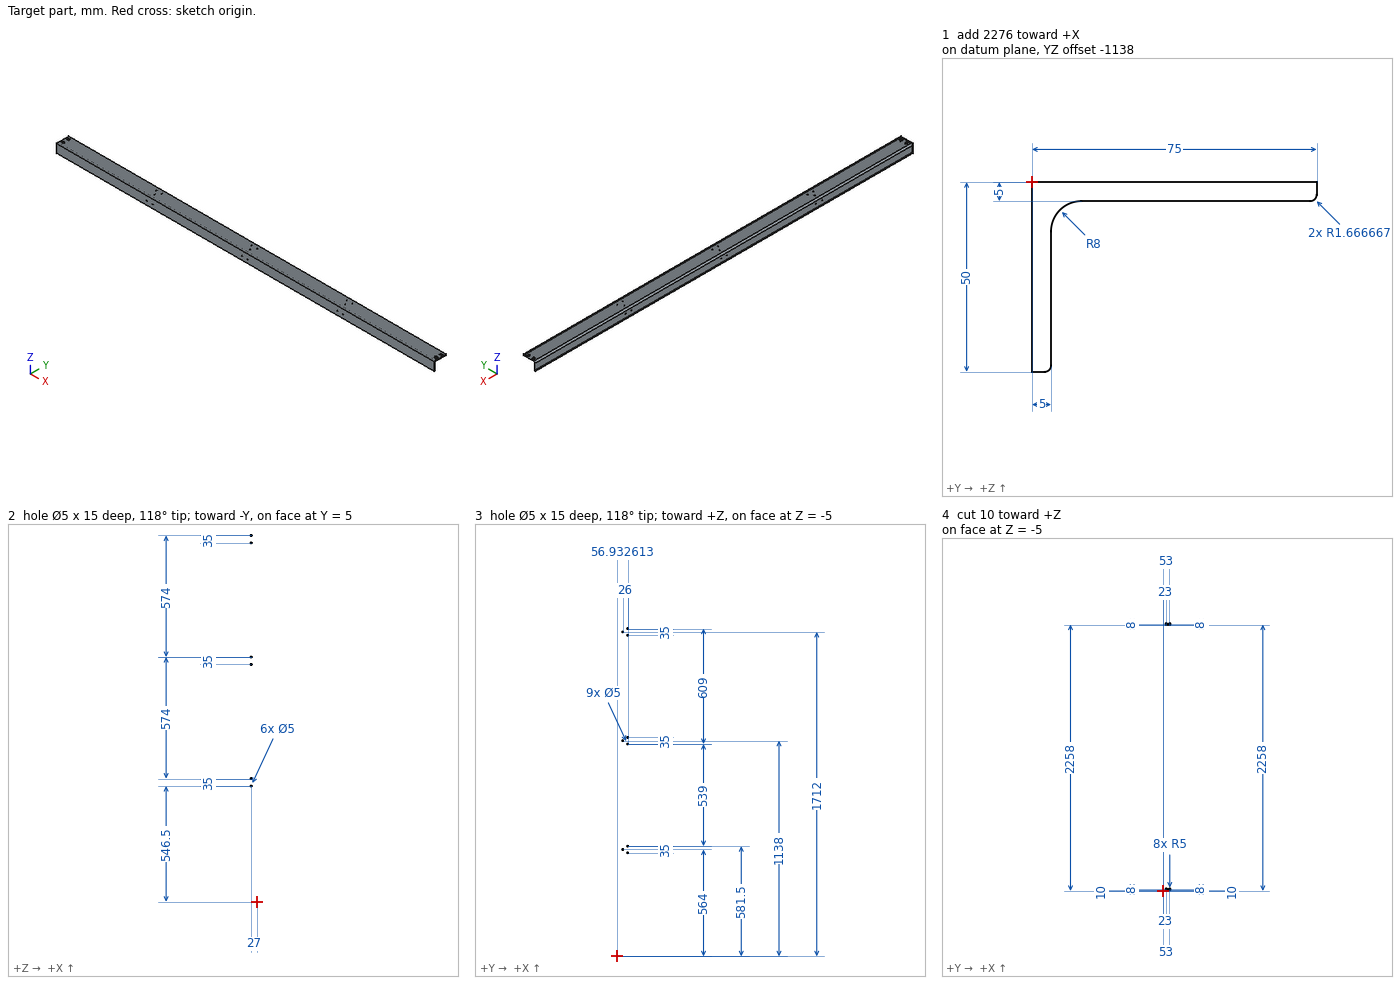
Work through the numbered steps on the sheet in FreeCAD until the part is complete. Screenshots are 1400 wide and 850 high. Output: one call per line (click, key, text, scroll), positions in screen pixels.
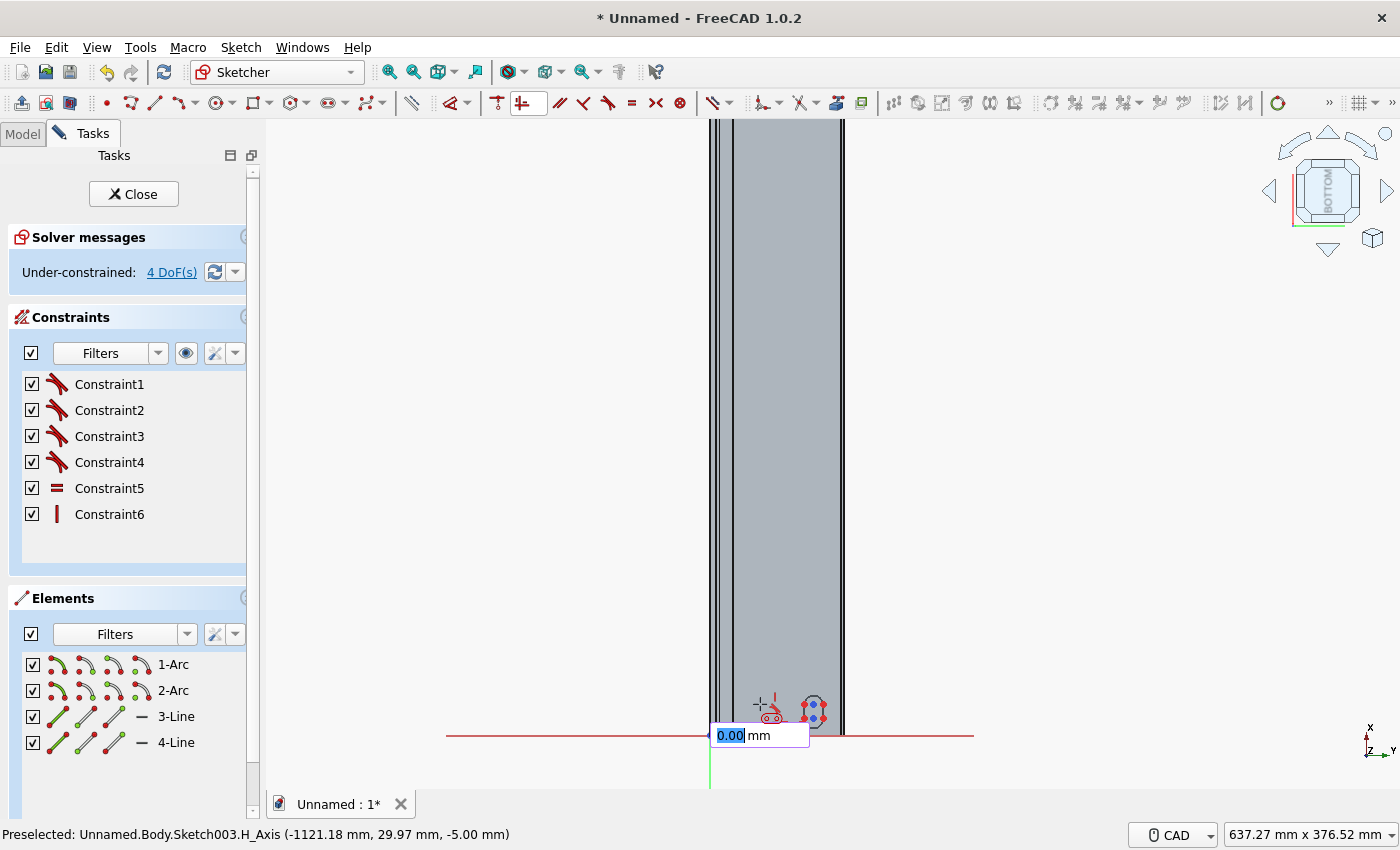
scroll(769, 711, up, 3)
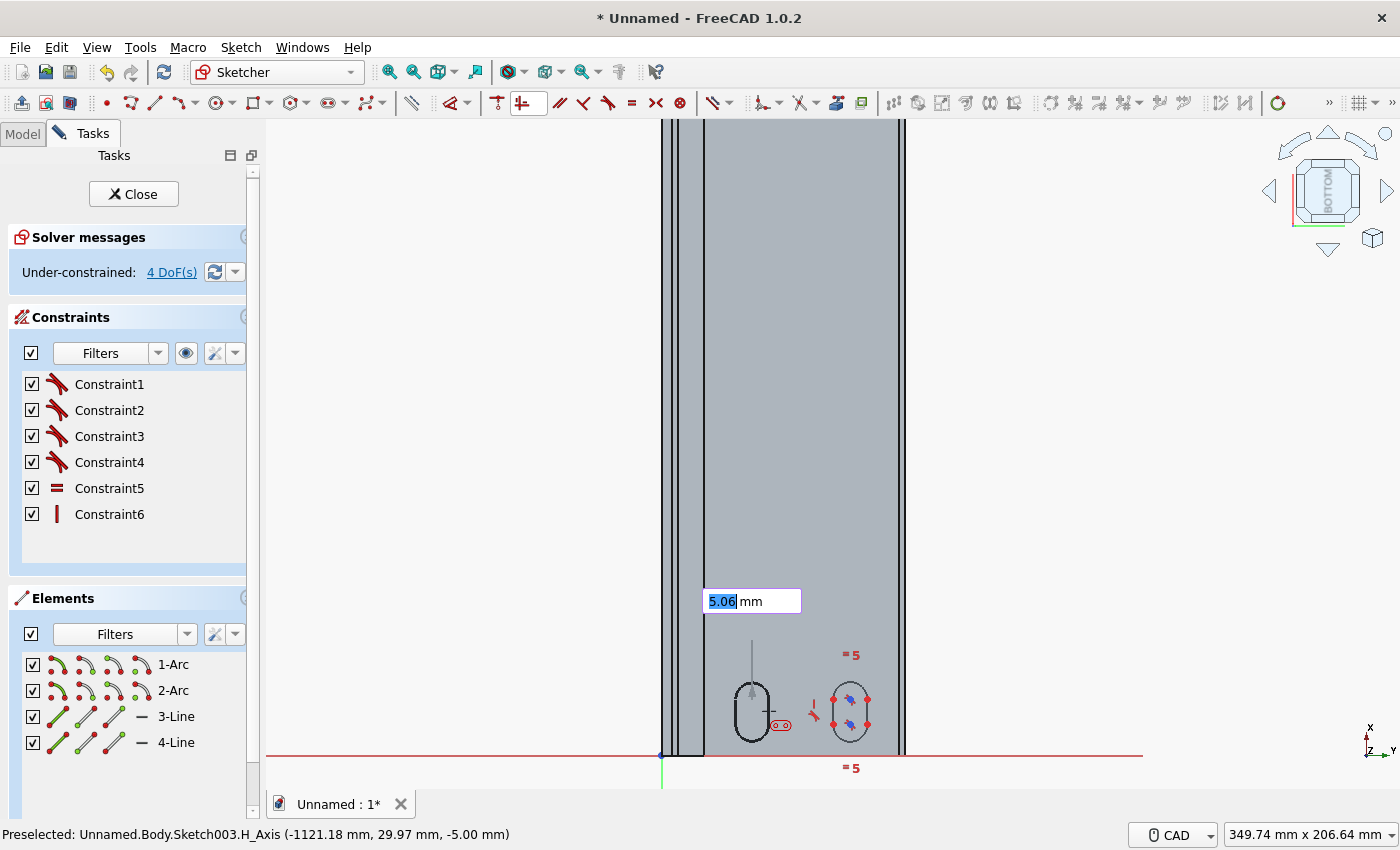
click(769, 710)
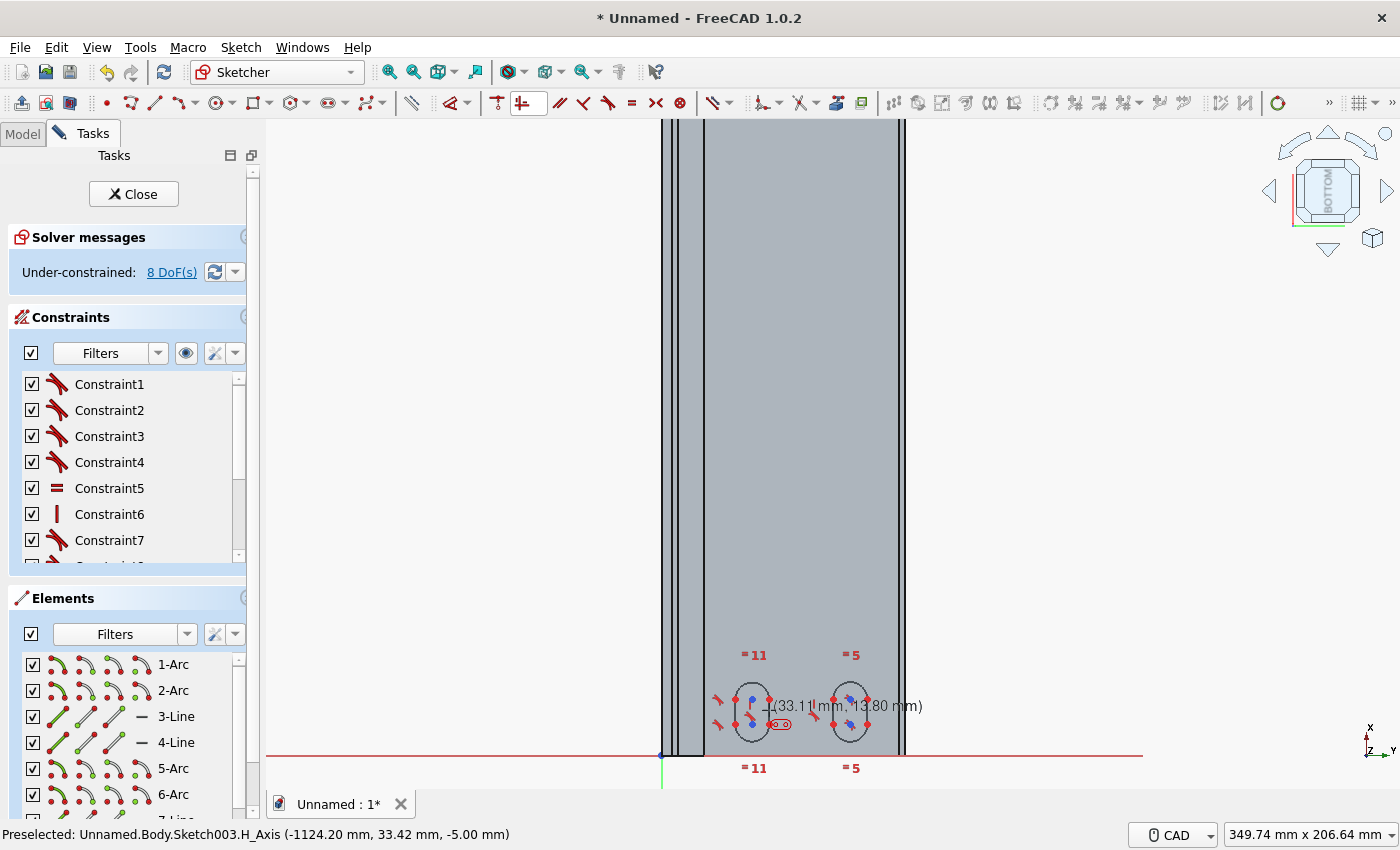
scroll(765, 673, down, 14)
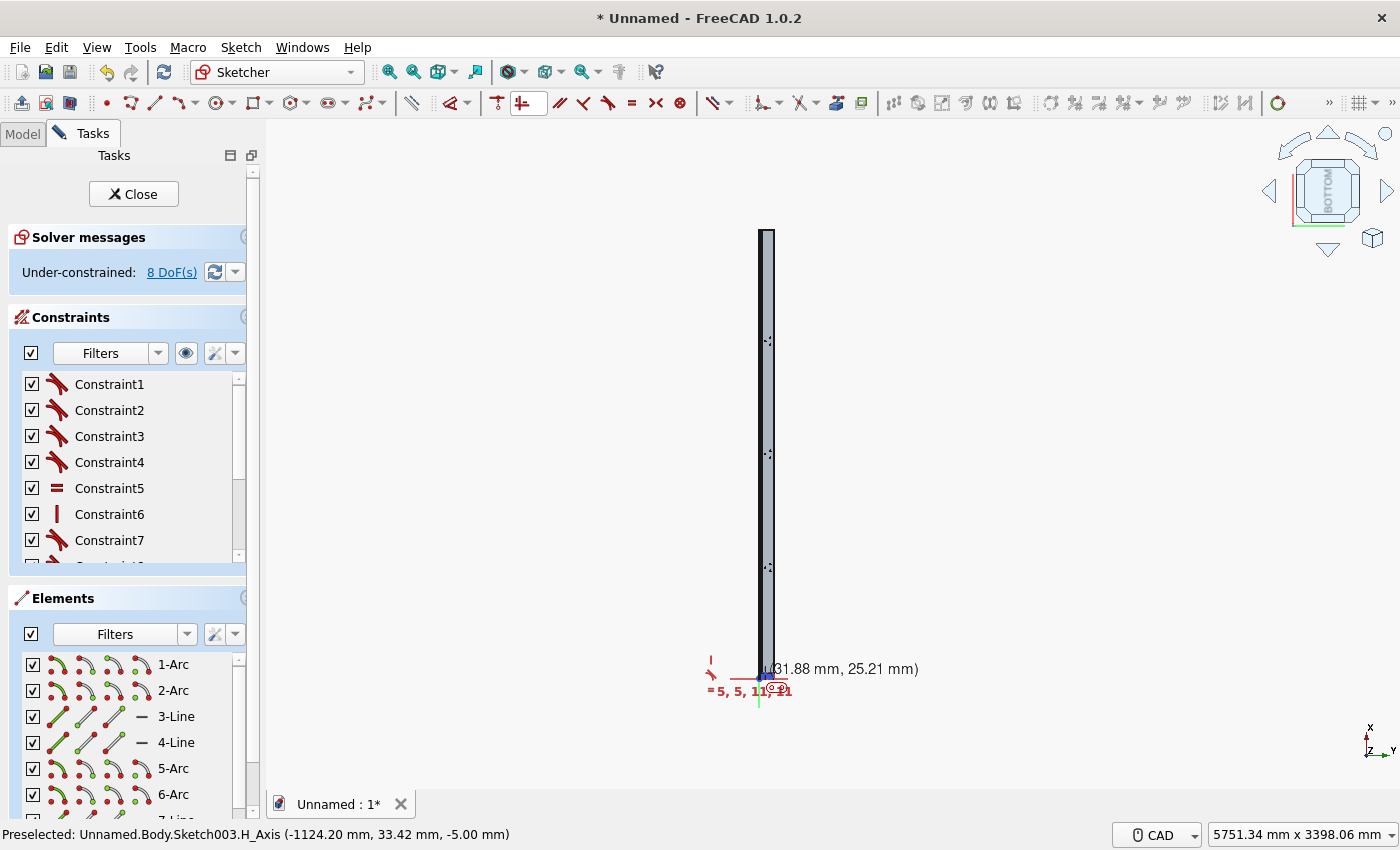
scroll(771, 234, up, 16)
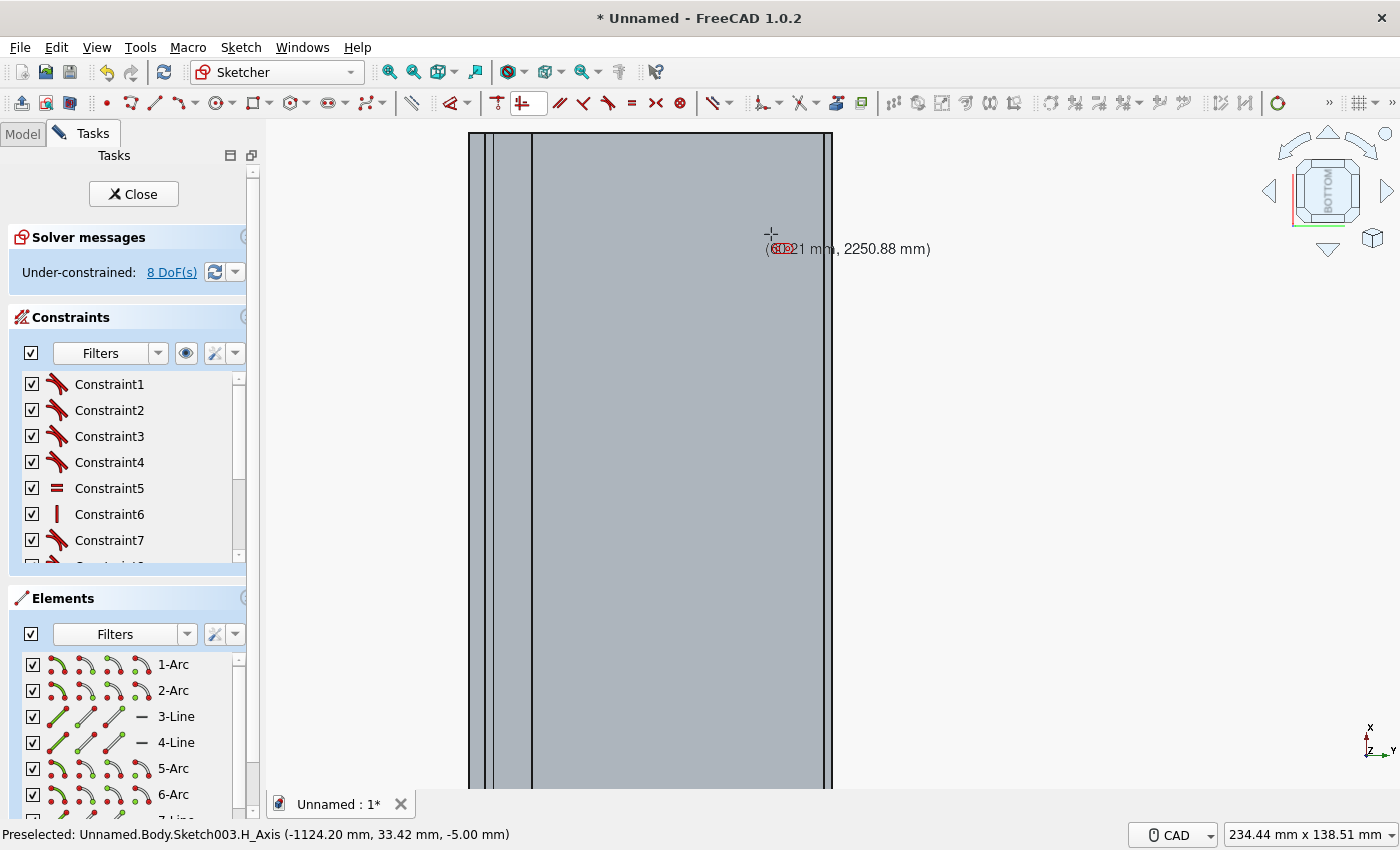
scroll(772, 182, down, 15)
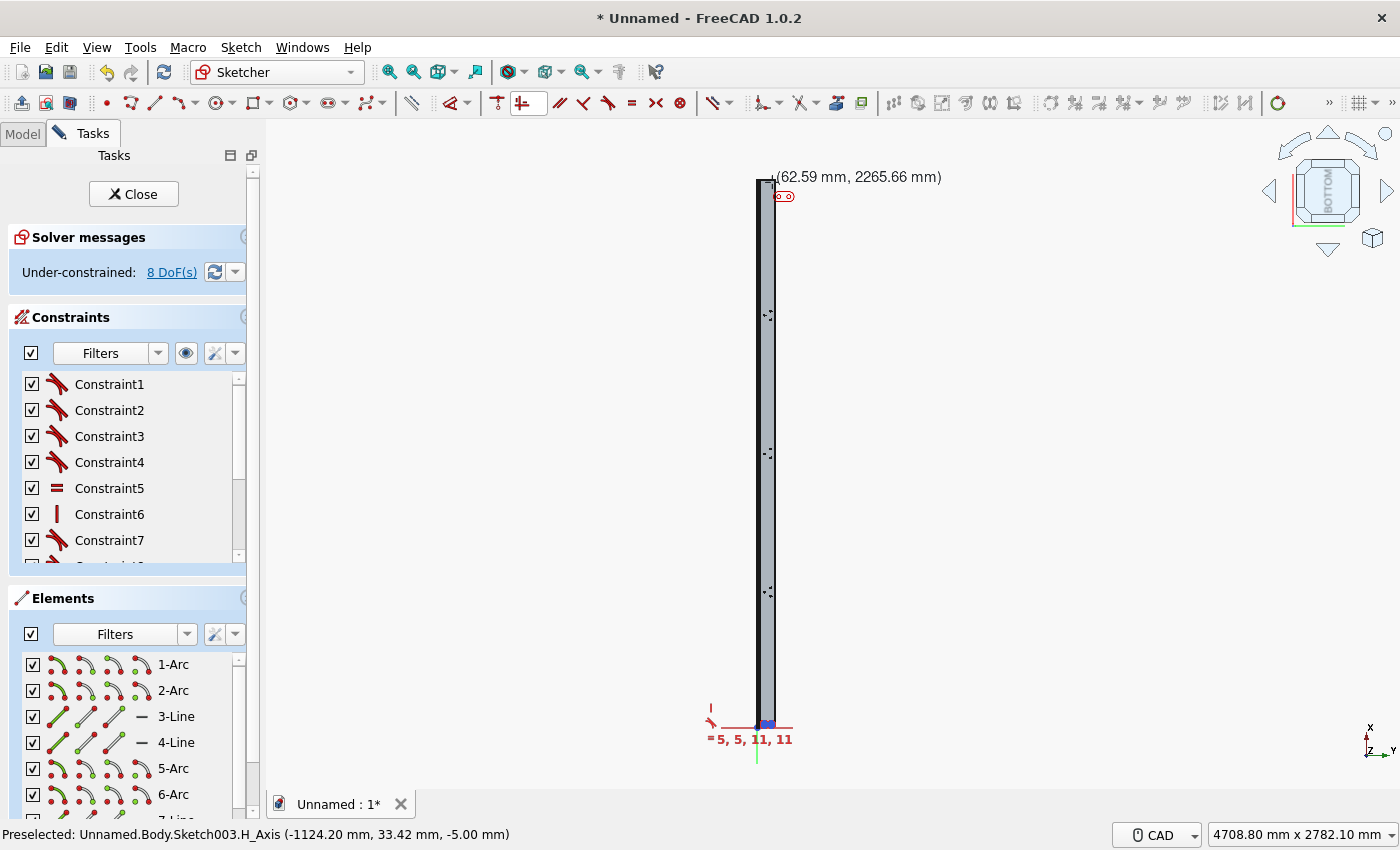
click(771, 184)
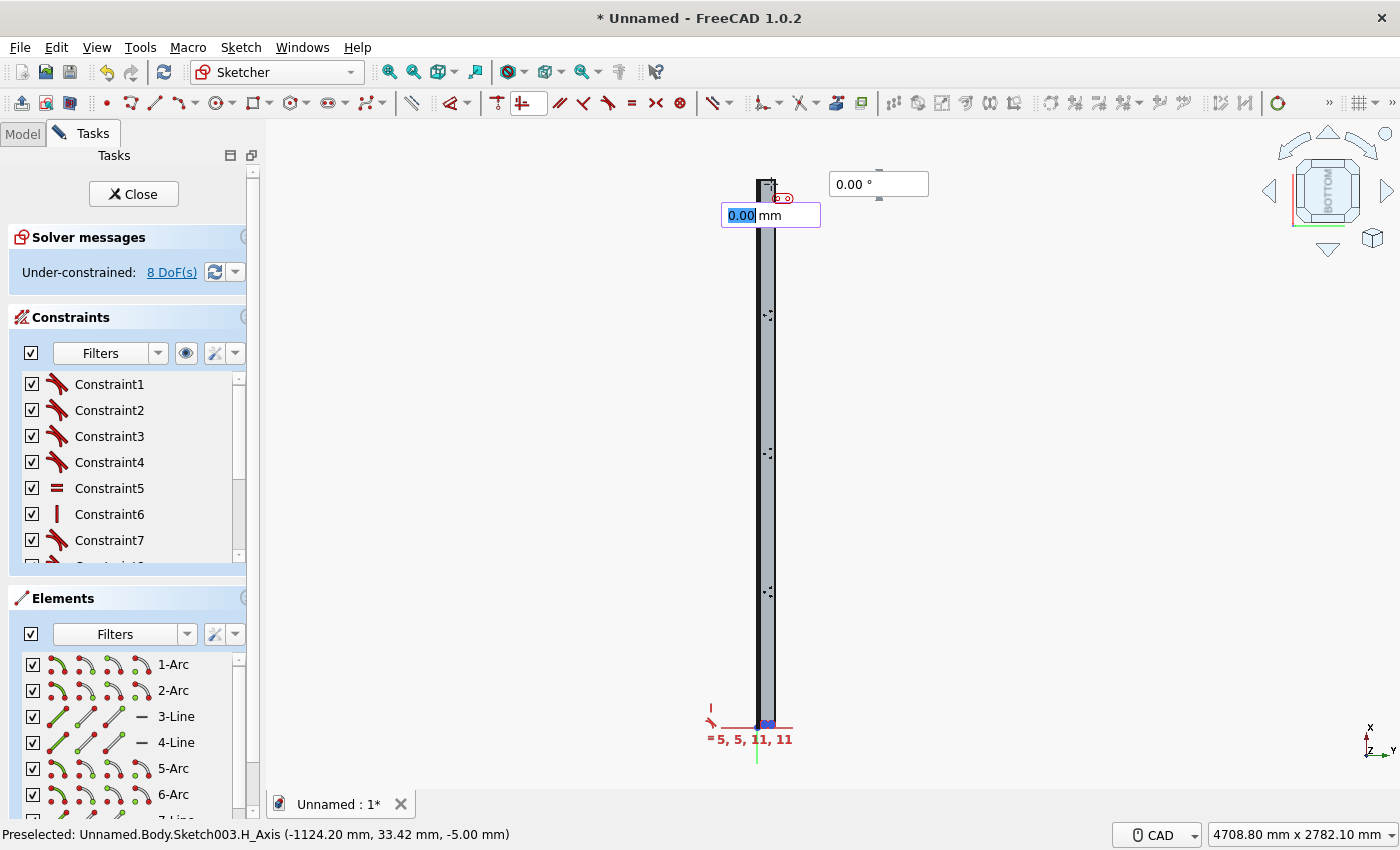
scroll(771, 182, up, 11)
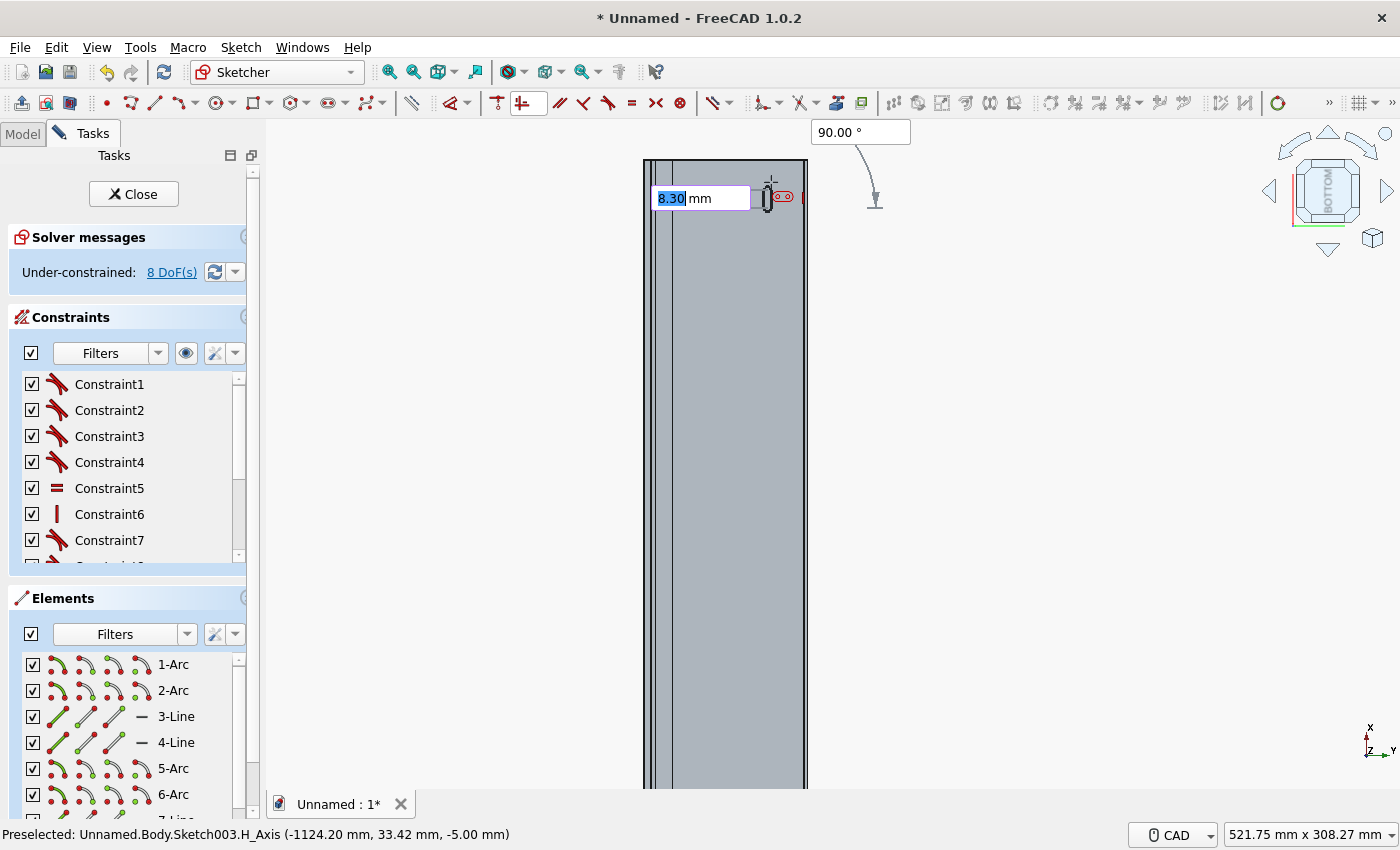
click(767, 182)